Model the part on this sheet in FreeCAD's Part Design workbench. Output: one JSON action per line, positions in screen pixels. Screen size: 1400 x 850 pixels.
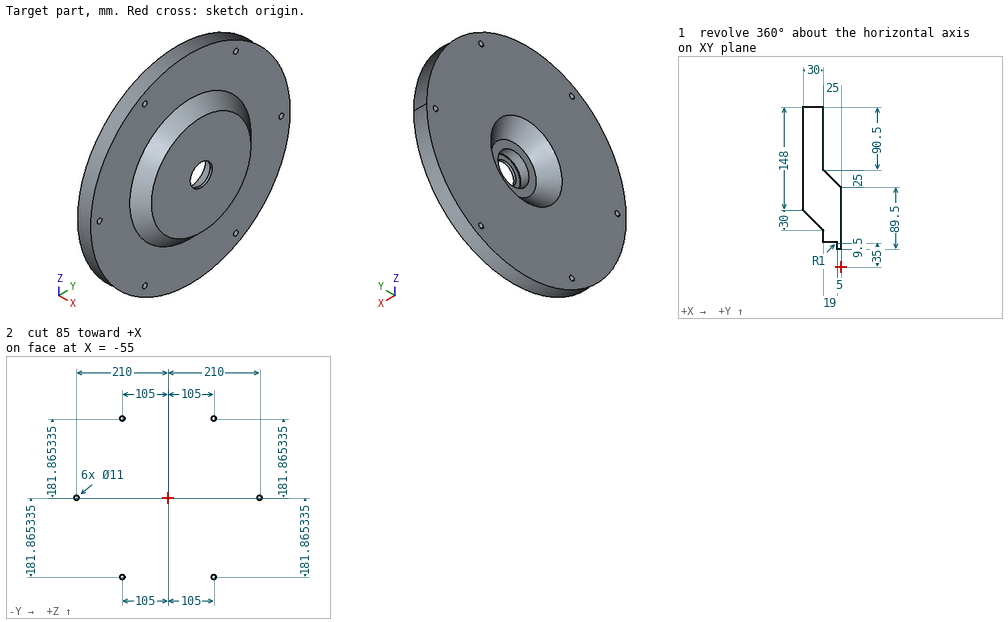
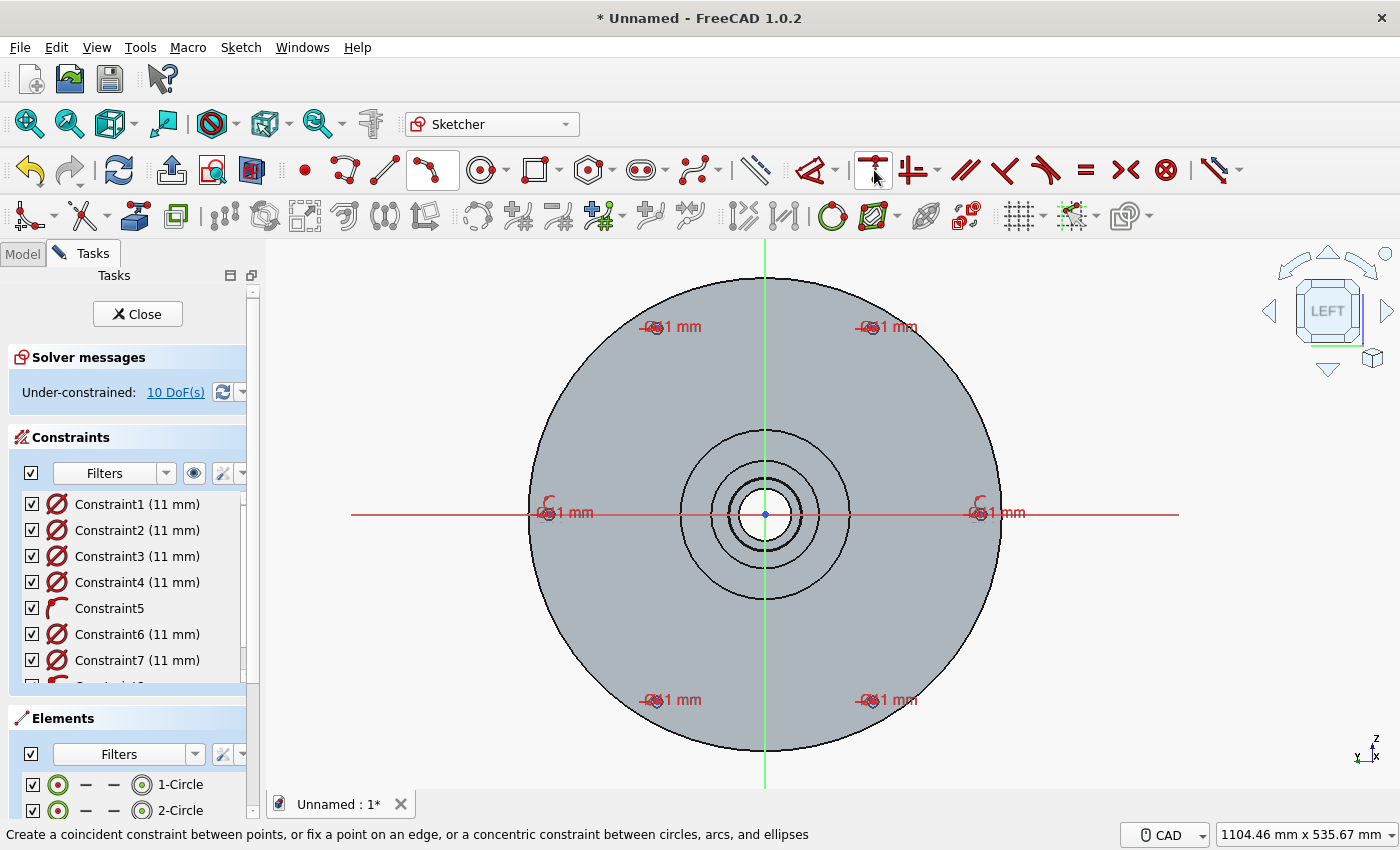
{"action": "left_click", "coordinate": [810, 170]}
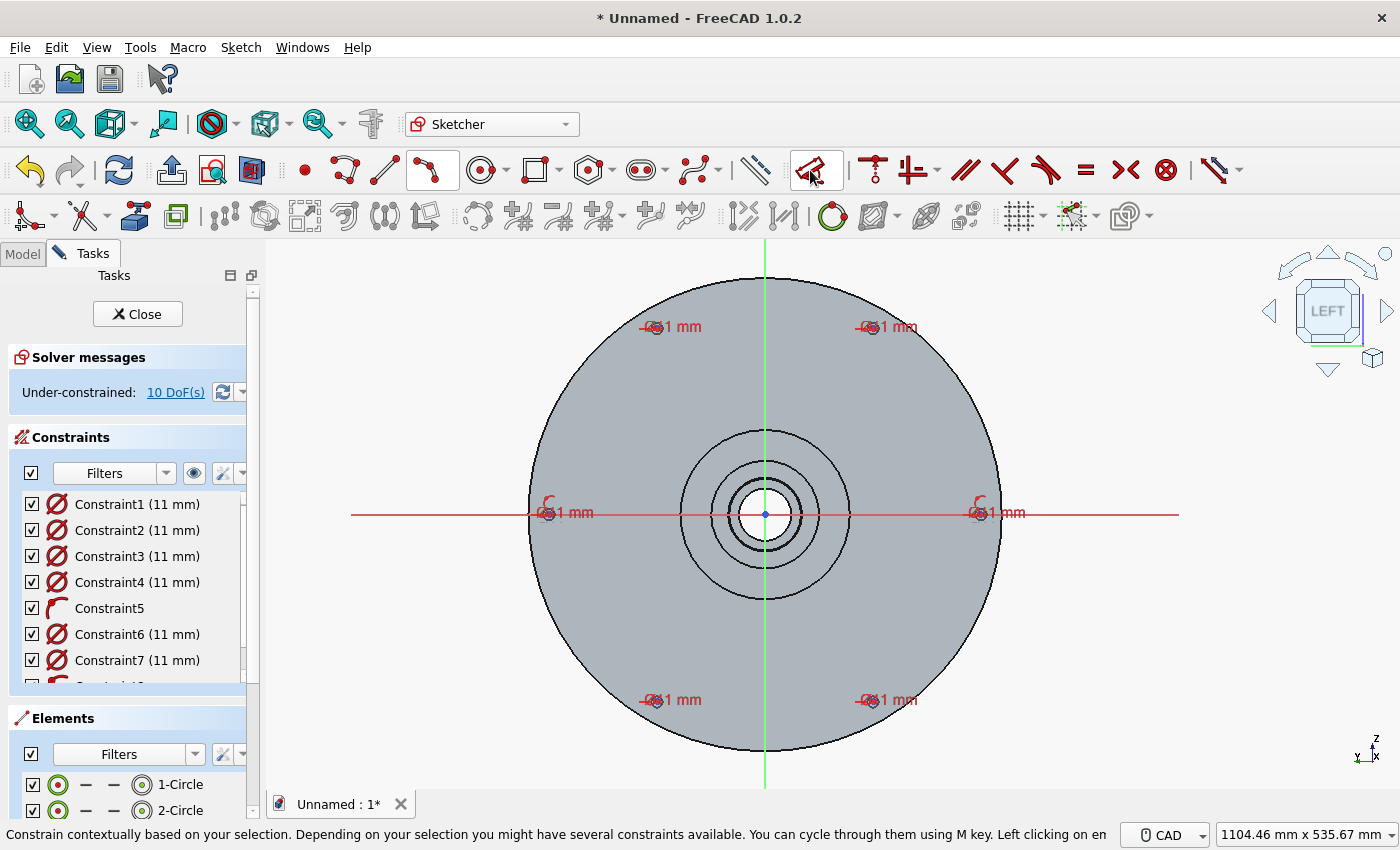
{"action": "left_click", "coordinate": [549, 515]}
{"action": "left_click", "coordinate": [657, 549]}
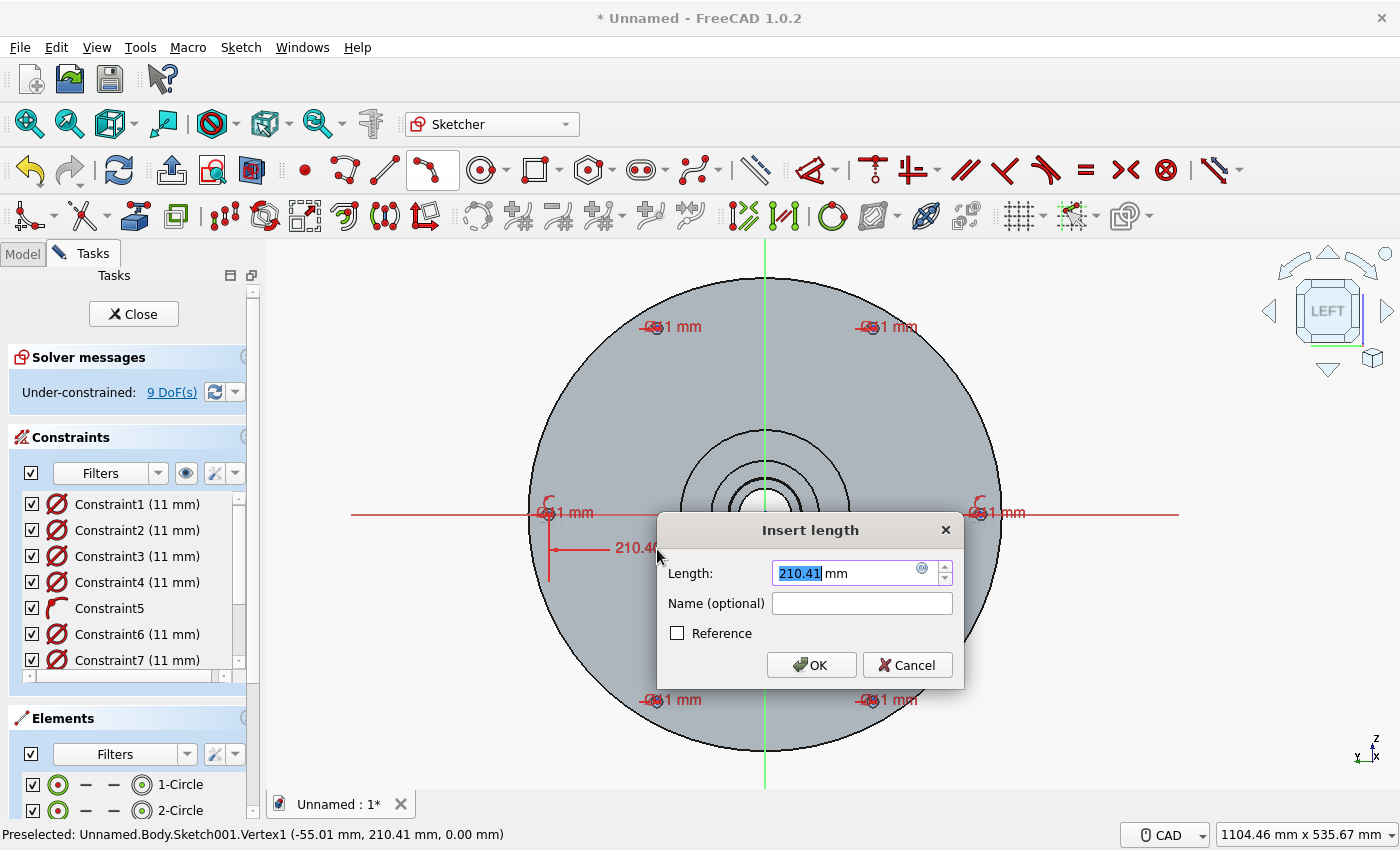
{"action": "type", "text": "210"}
{"action": "key", "text": "Return"}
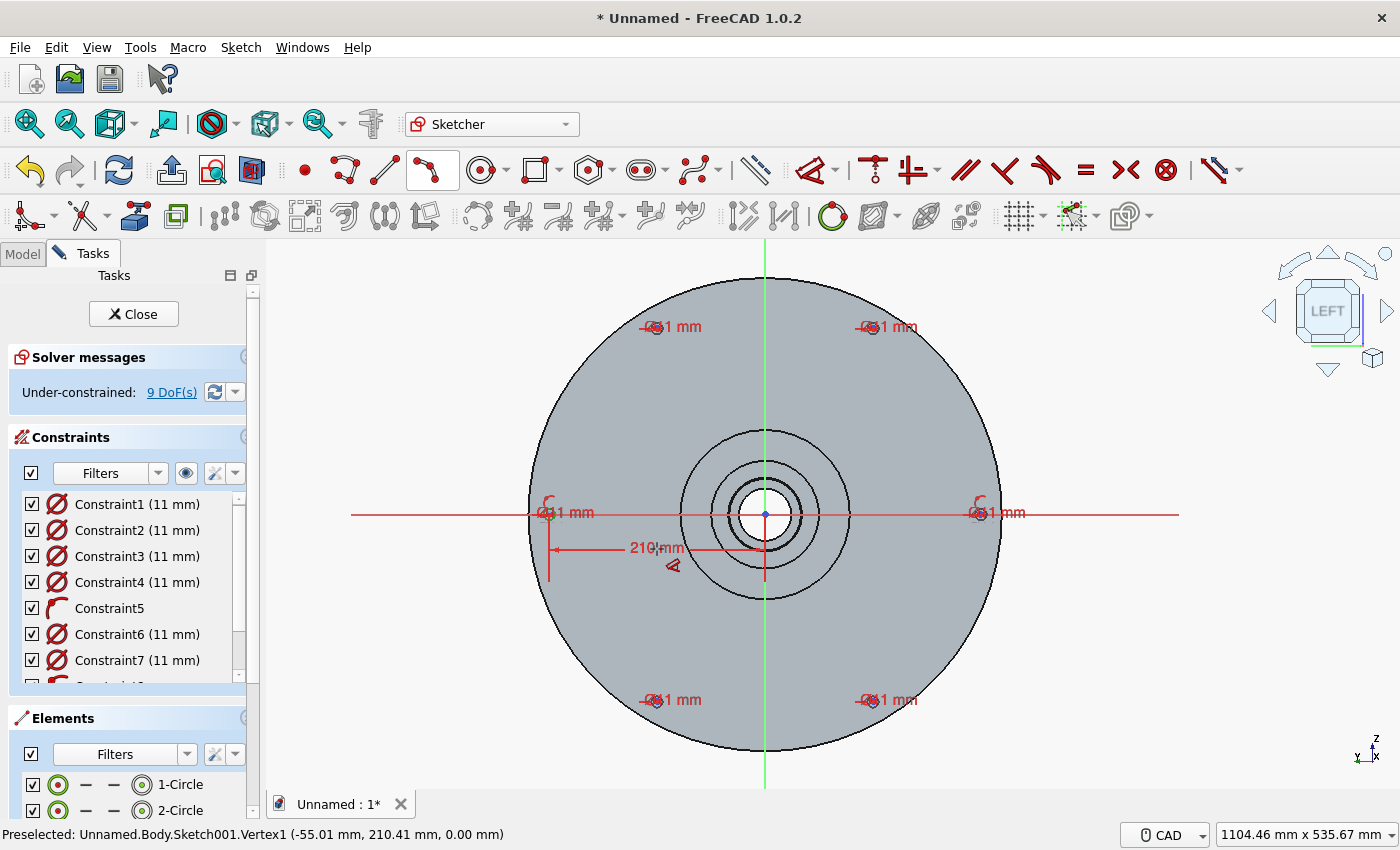
{"action": "left_click", "coordinate": [657, 329]}
{"action": "left_click", "coordinate": [711, 295]}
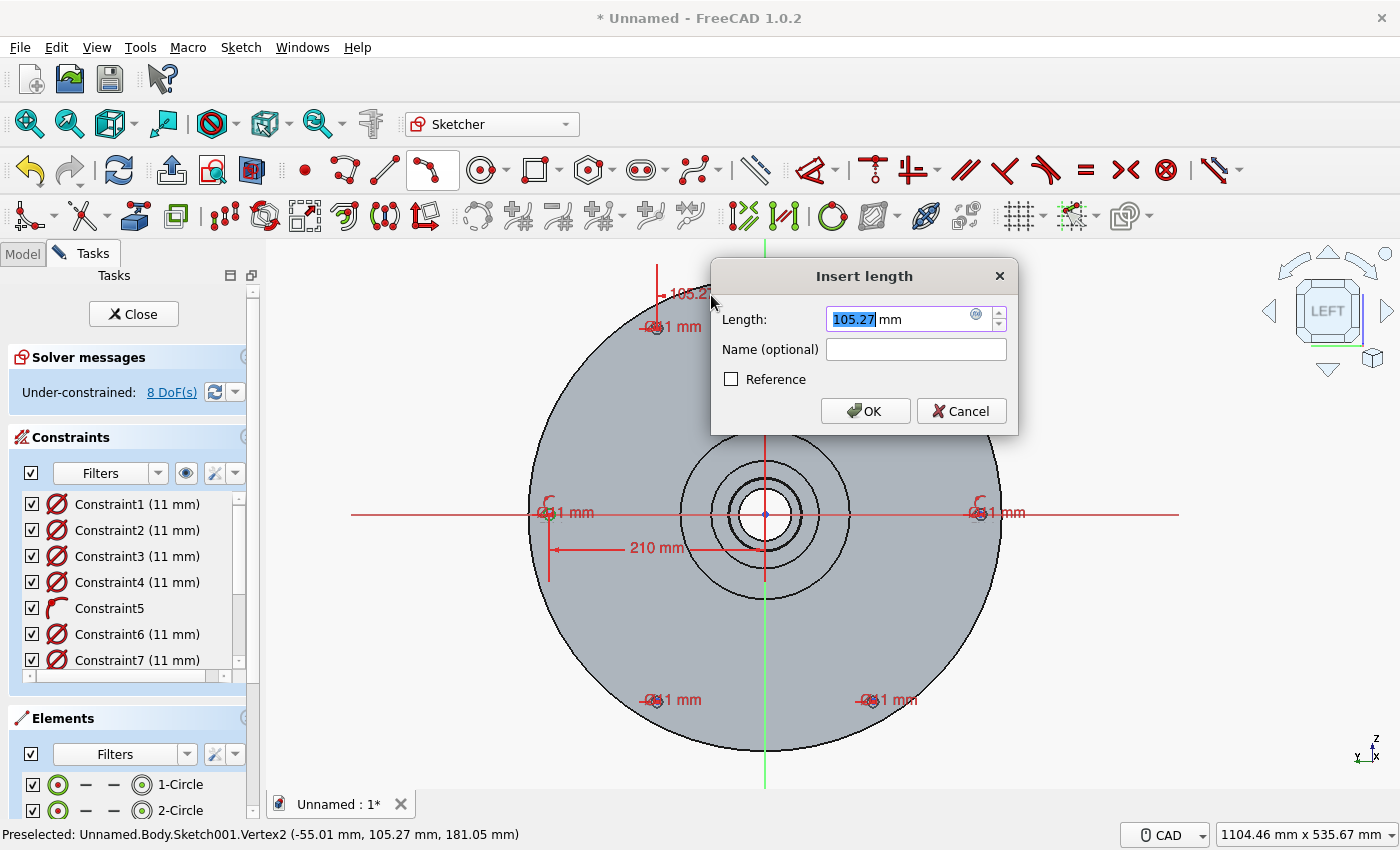
{"action": "type", "text": "105"}
{"action": "key", "text": "Return"}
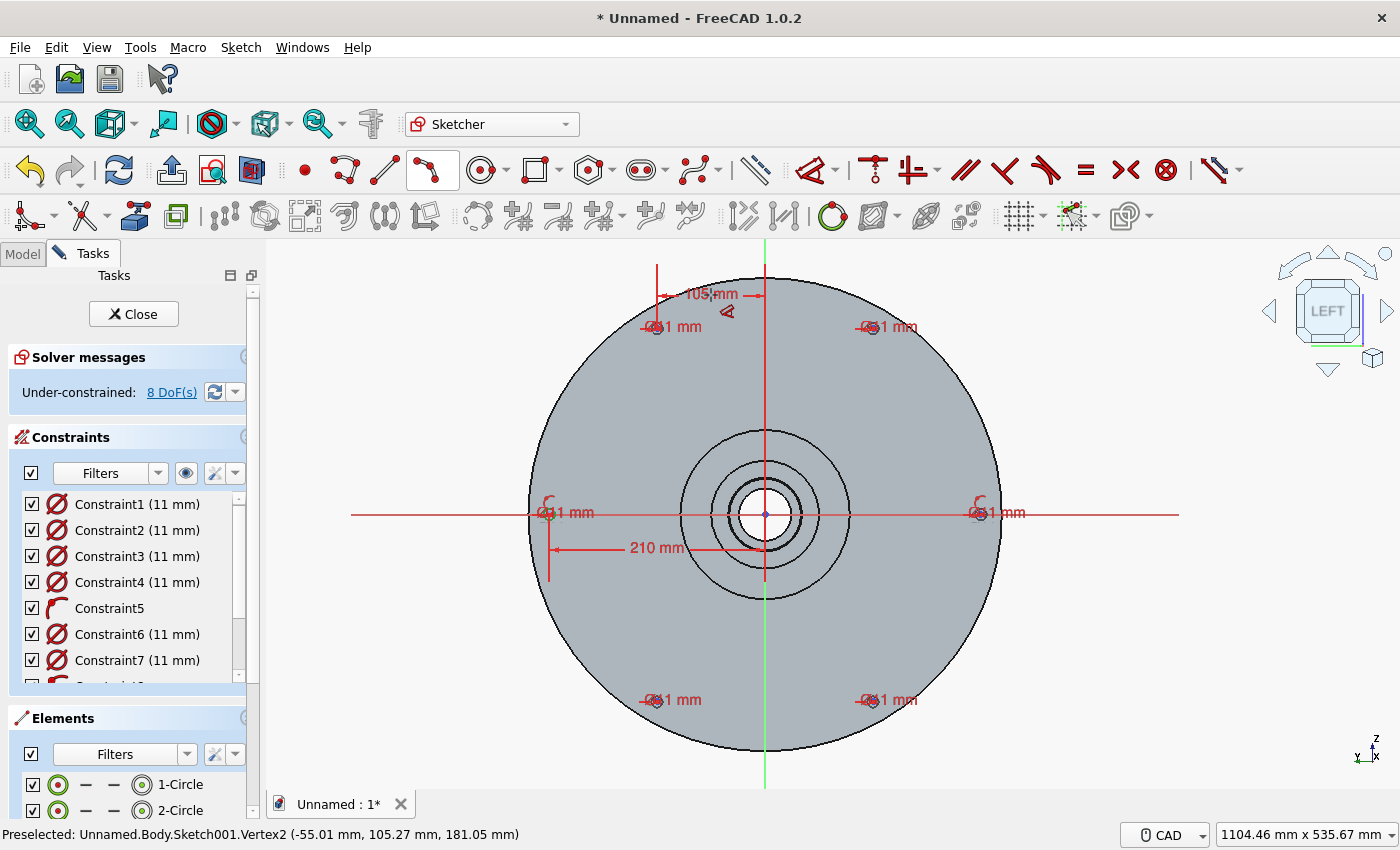
{"action": "left_click", "coordinate": [873, 329]}
{"action": "left_click", "coordinate": [819, 295]}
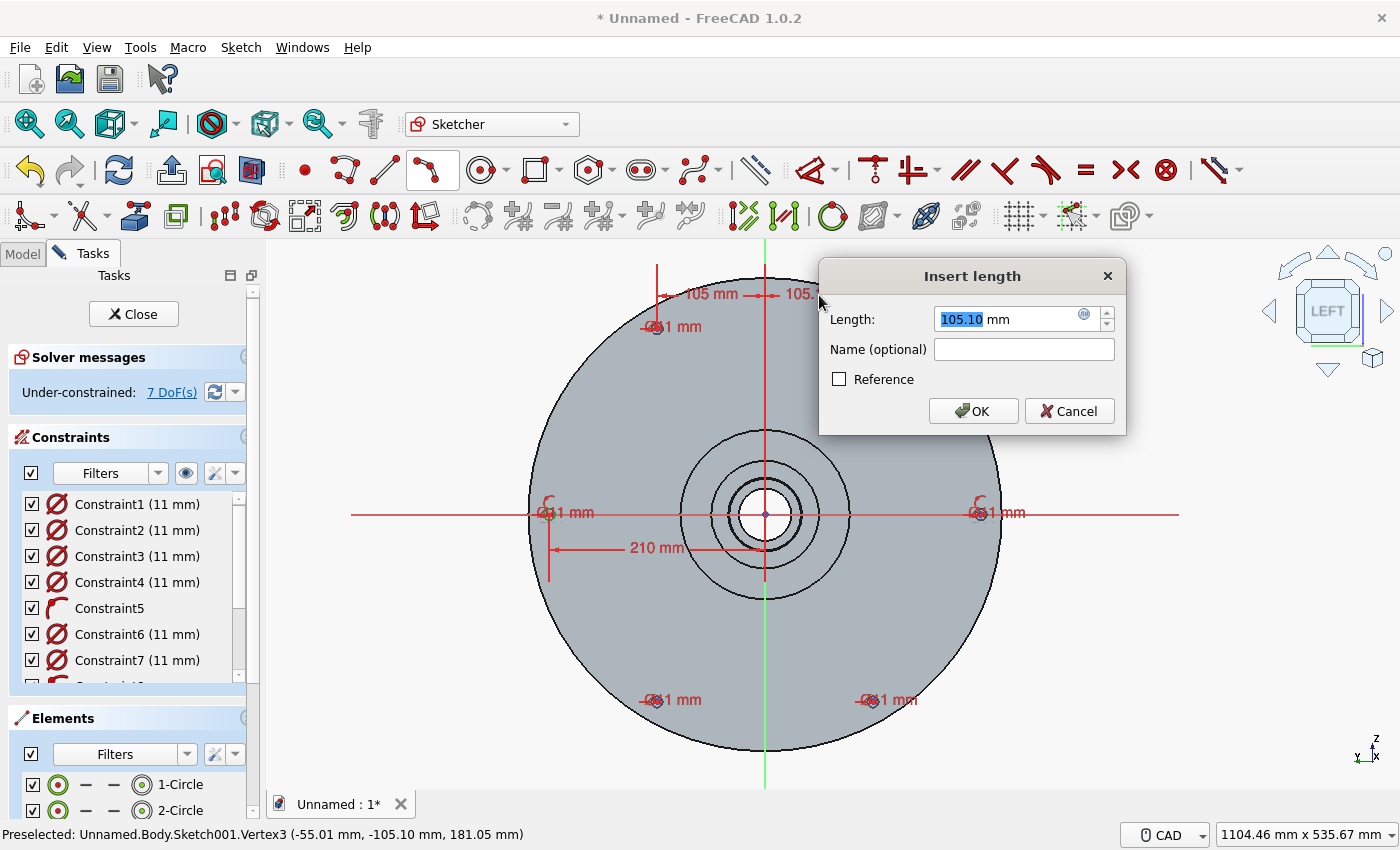
{"action": "type", "text": "105"}
{"action": "key", "text": "Return"}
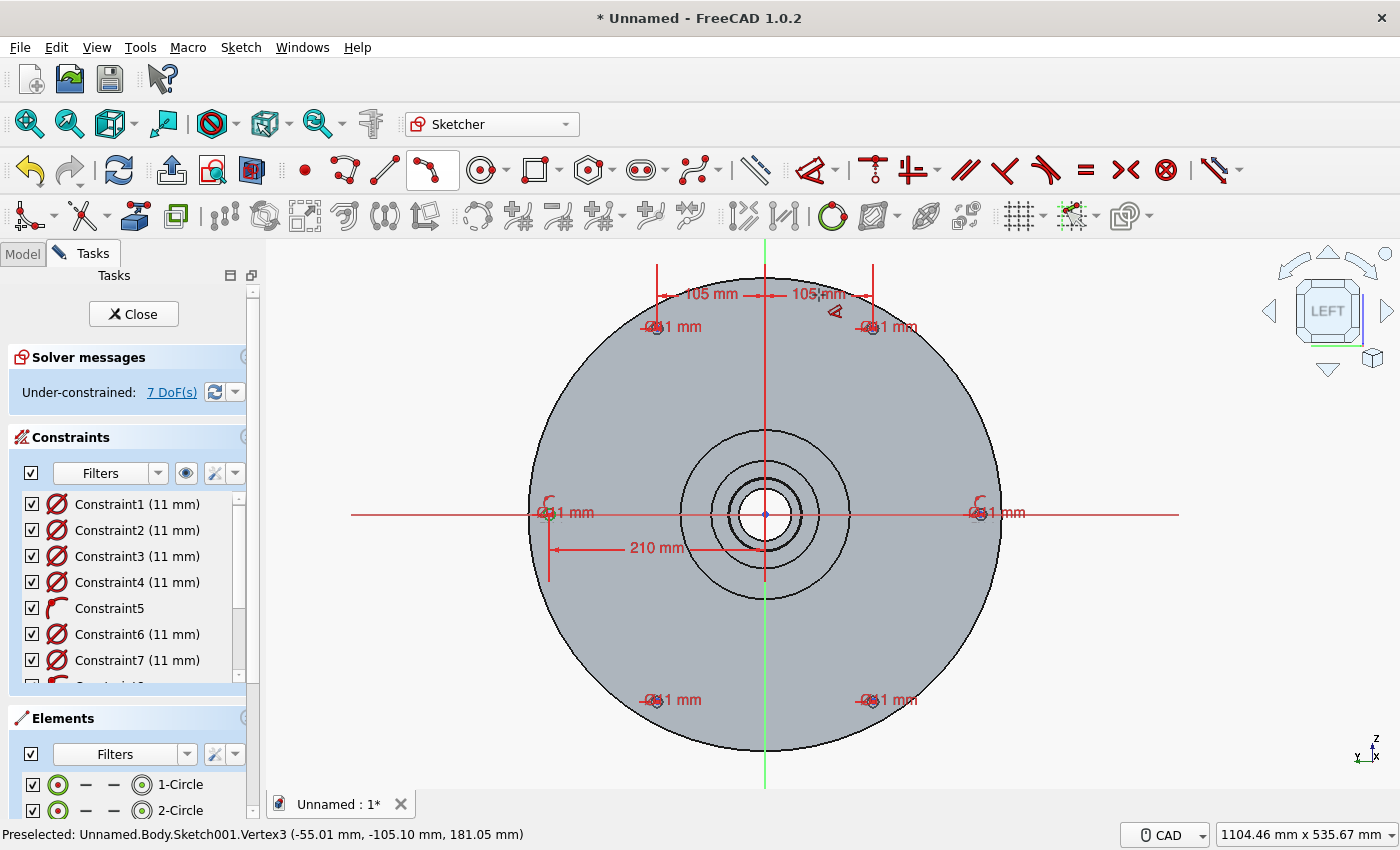
{"action": "left_click", "coordinate": [981, 515]}
{"action": "left_click", "coordinate": [873, 549]}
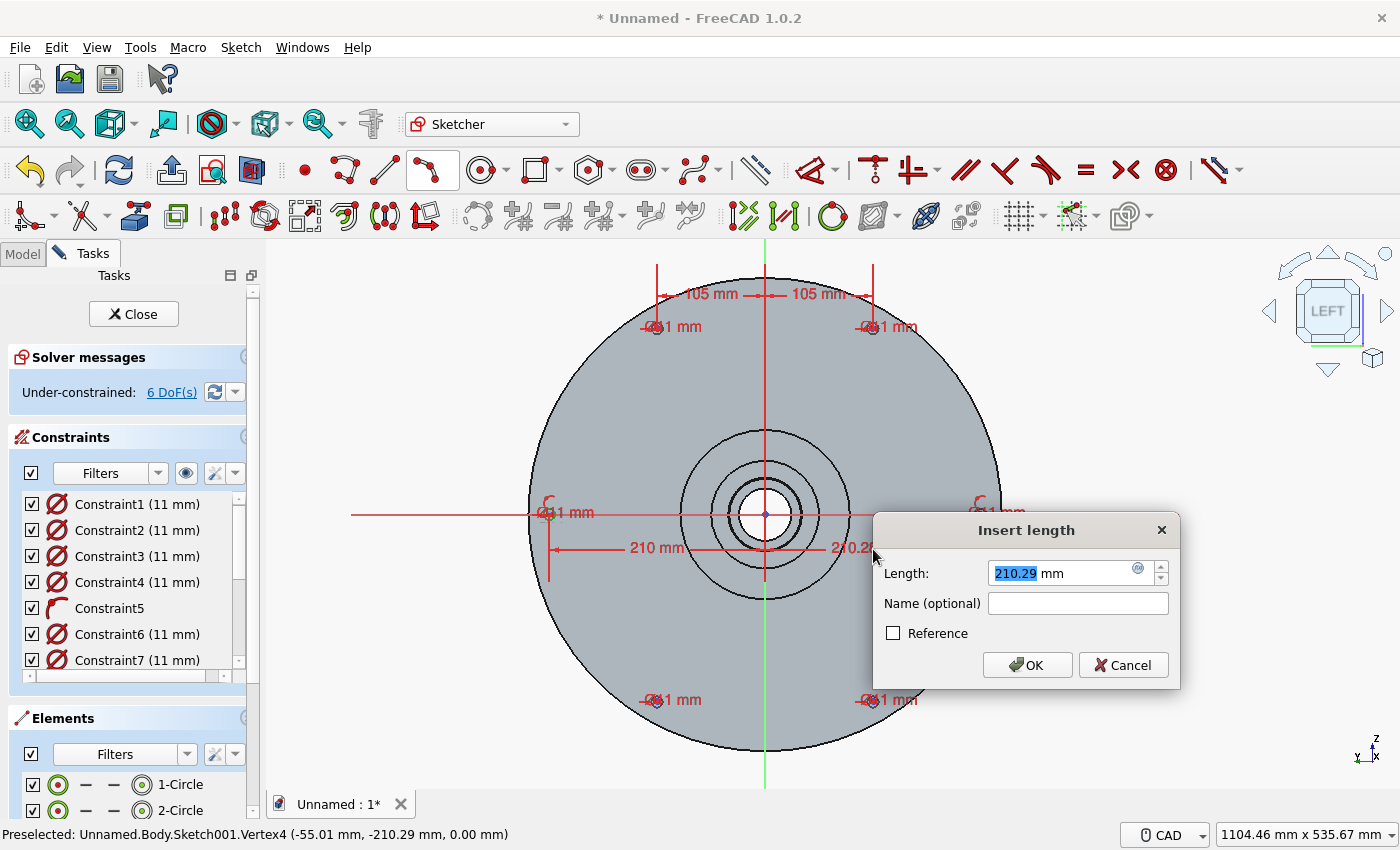
{"action": "type", "text": "210"}
{"action": "key", "text": "Return"}